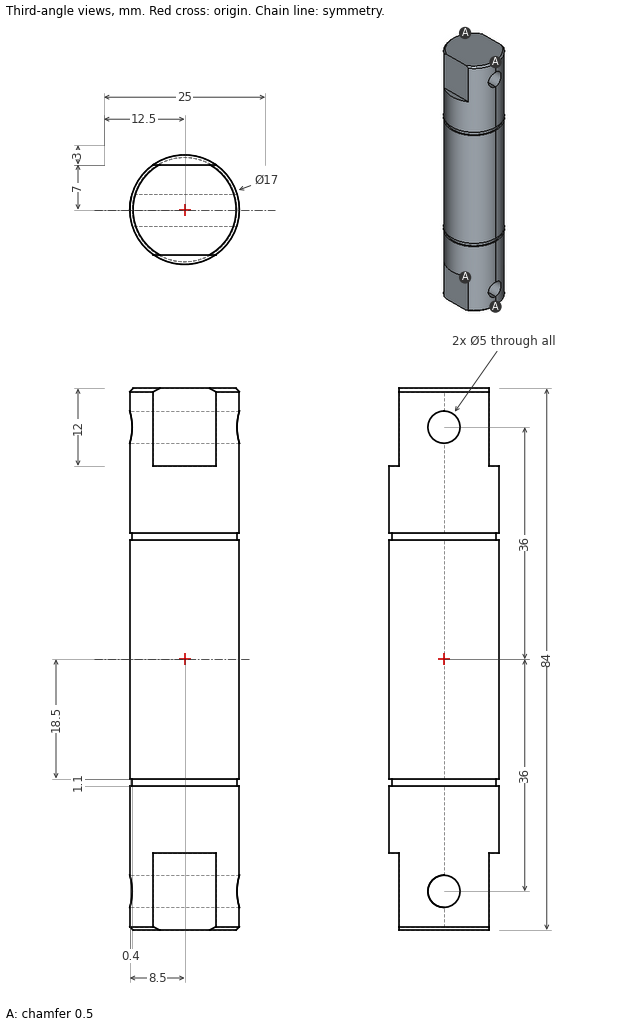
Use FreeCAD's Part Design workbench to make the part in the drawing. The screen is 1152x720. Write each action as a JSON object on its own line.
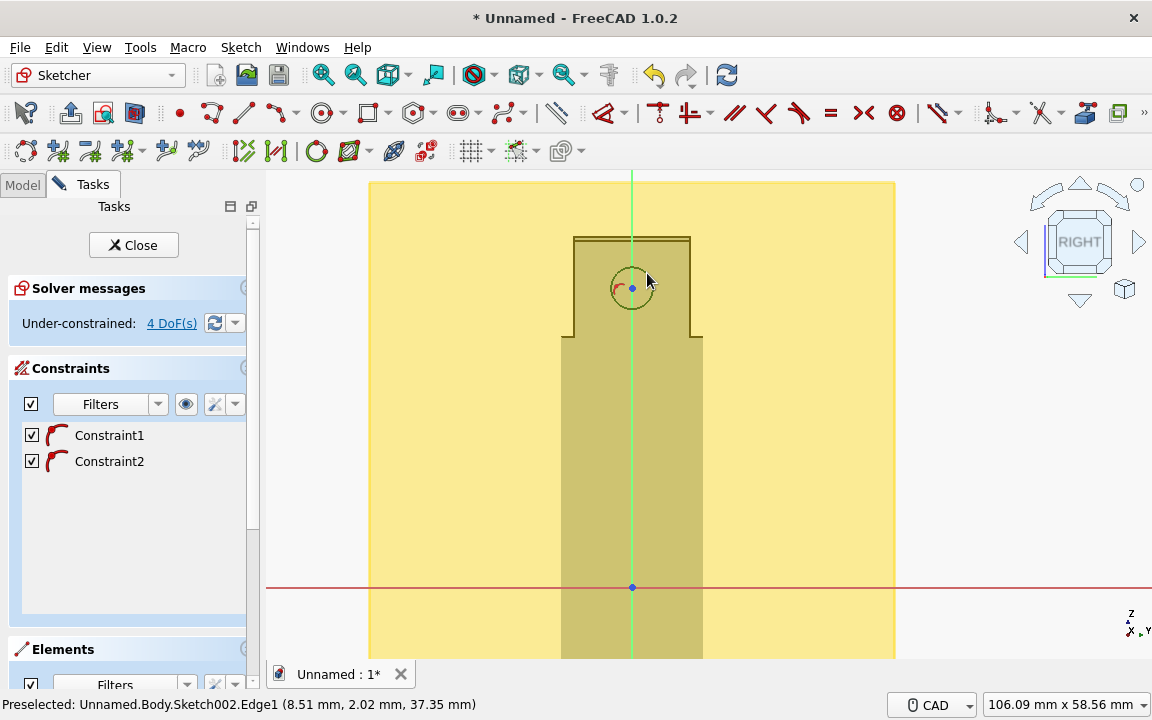
{"action": "scroll", "coordinate": [647, 273], "scroll_direction": "down", "scroll_amount": 4}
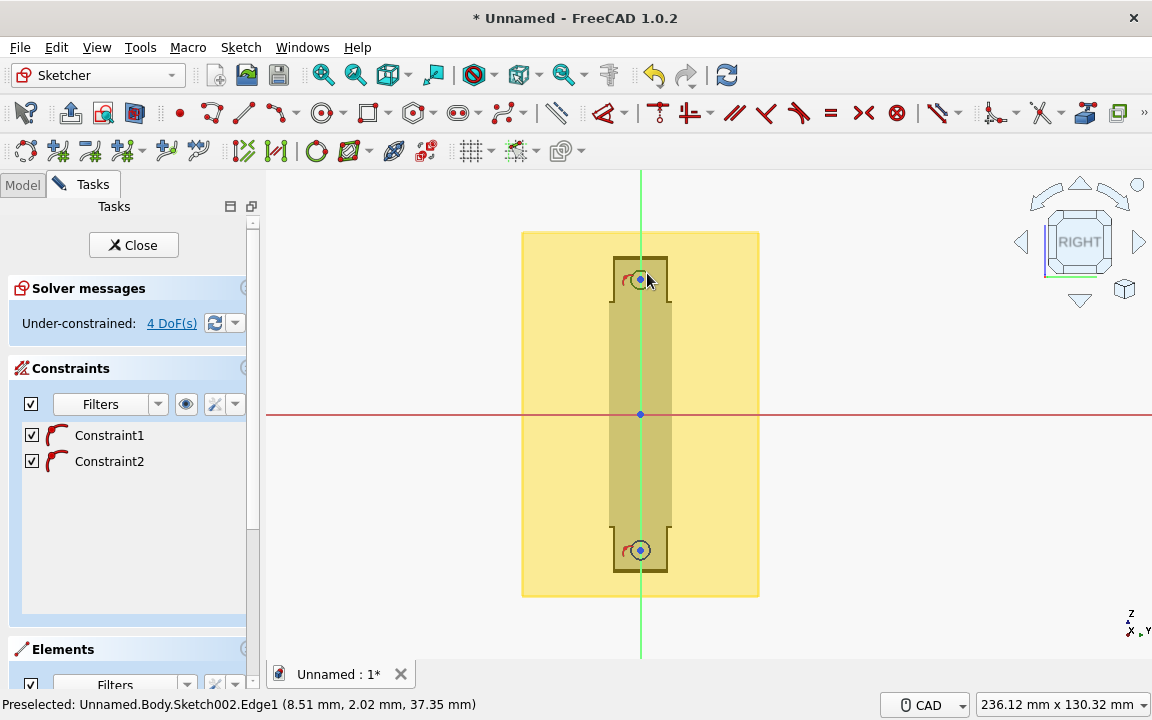
{"action": "scroll", "coordinate": [647, 544], "scroll_direction": "up", "scroll_amount": 4}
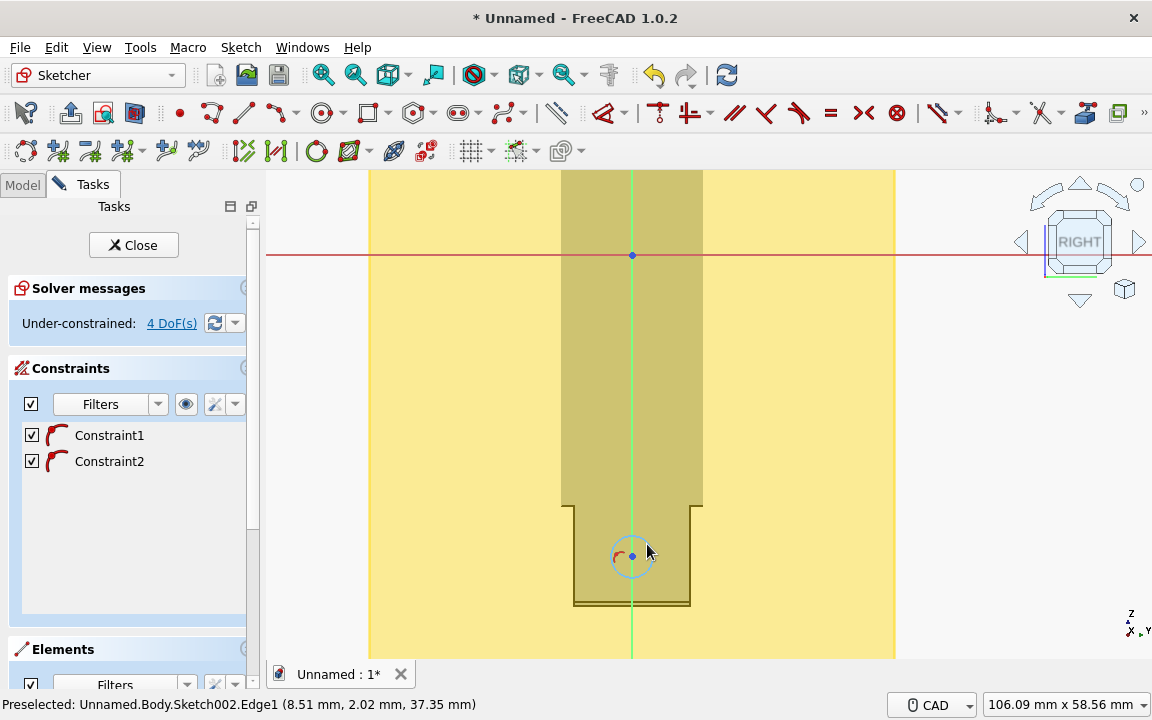
{"action": "left_click", "coordinate": [647, 542]}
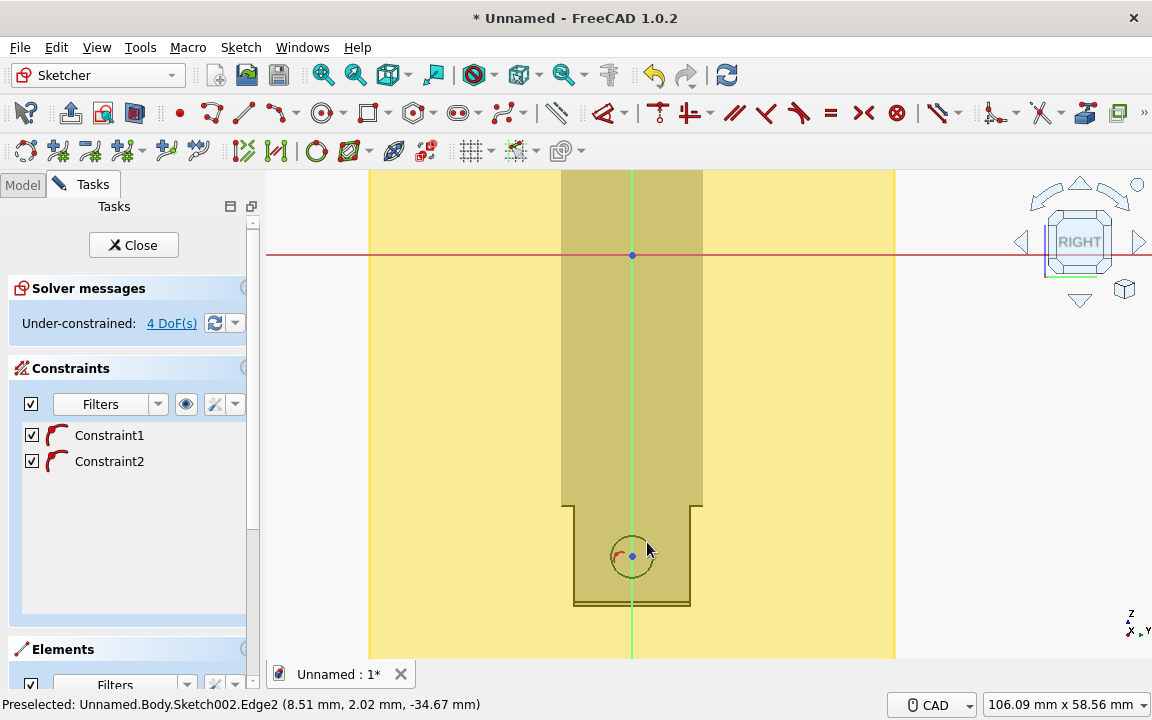
{"action": "left_click", "coordinate": [832, 114]}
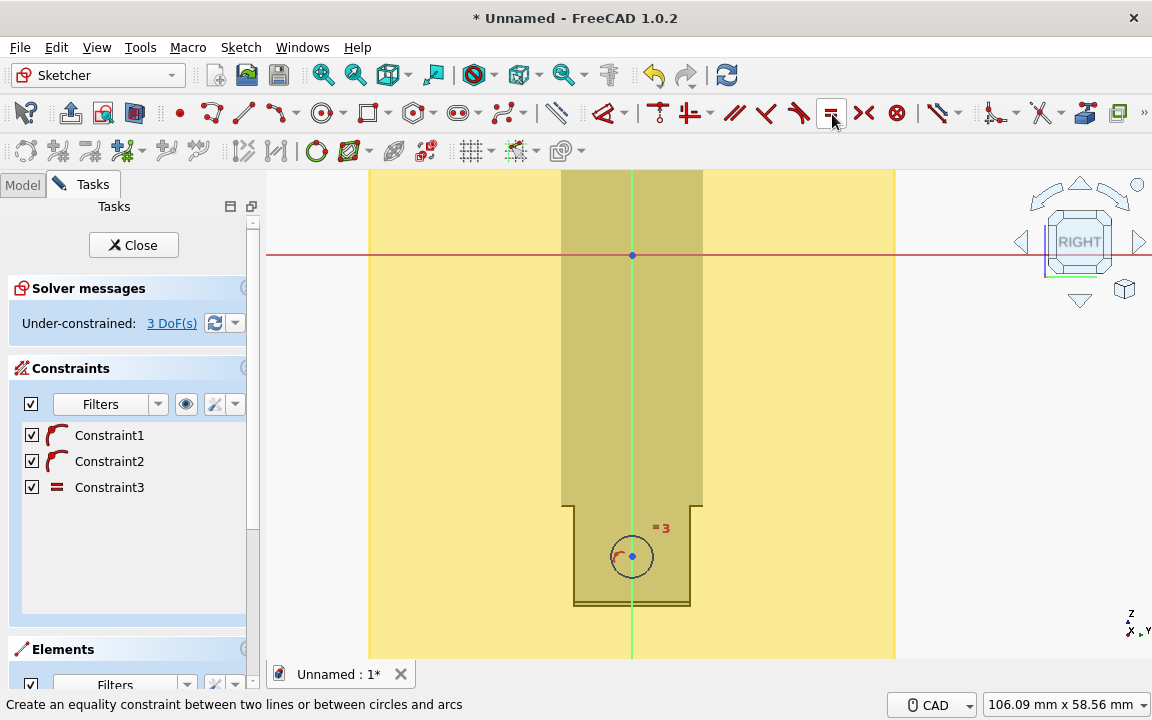
{"action": "left_click", "coordinate": [604, 114]}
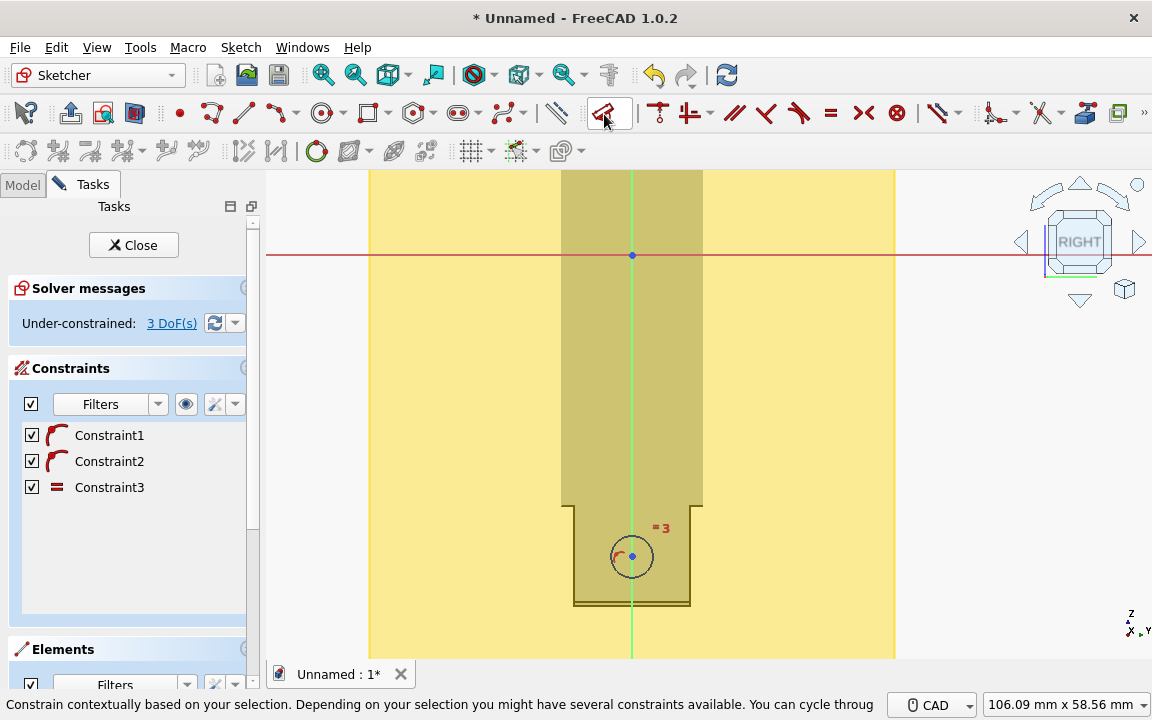
{"action": "scroll", "coordinate": [647, 545], "scroll_direction": "down", "scroll_amount": 4}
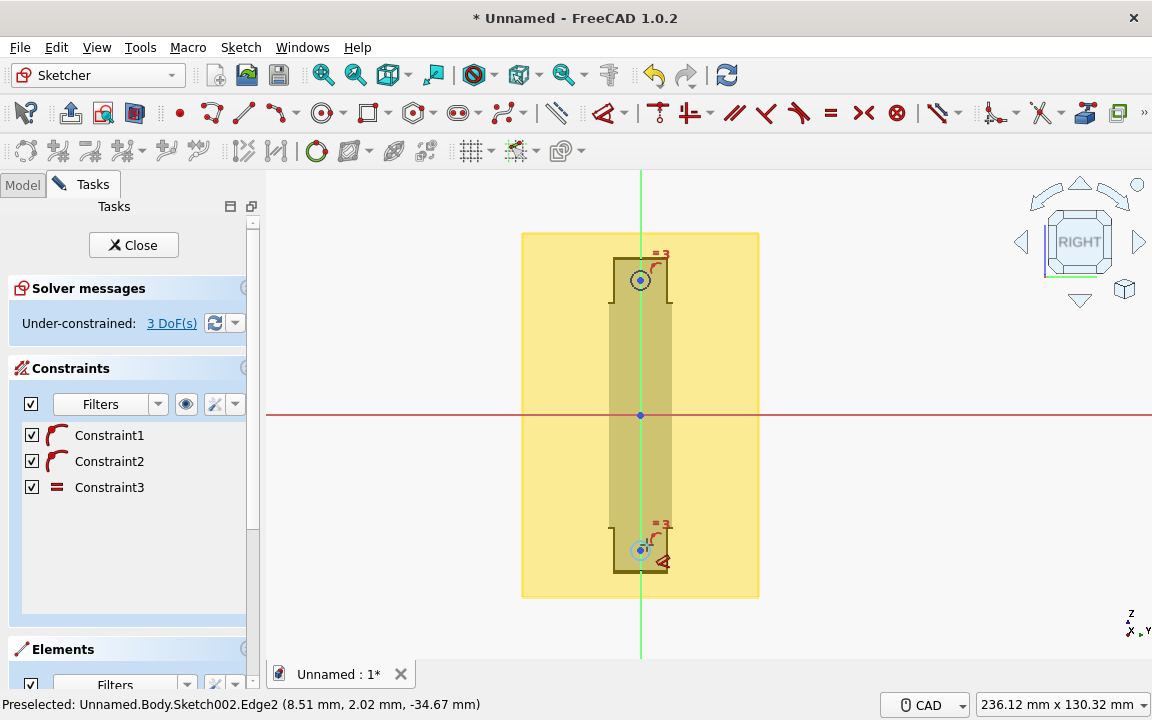
{"action": "scroll", "coordinate": [647, 274], "scroll_direction": "up", "scroll_amount": 4}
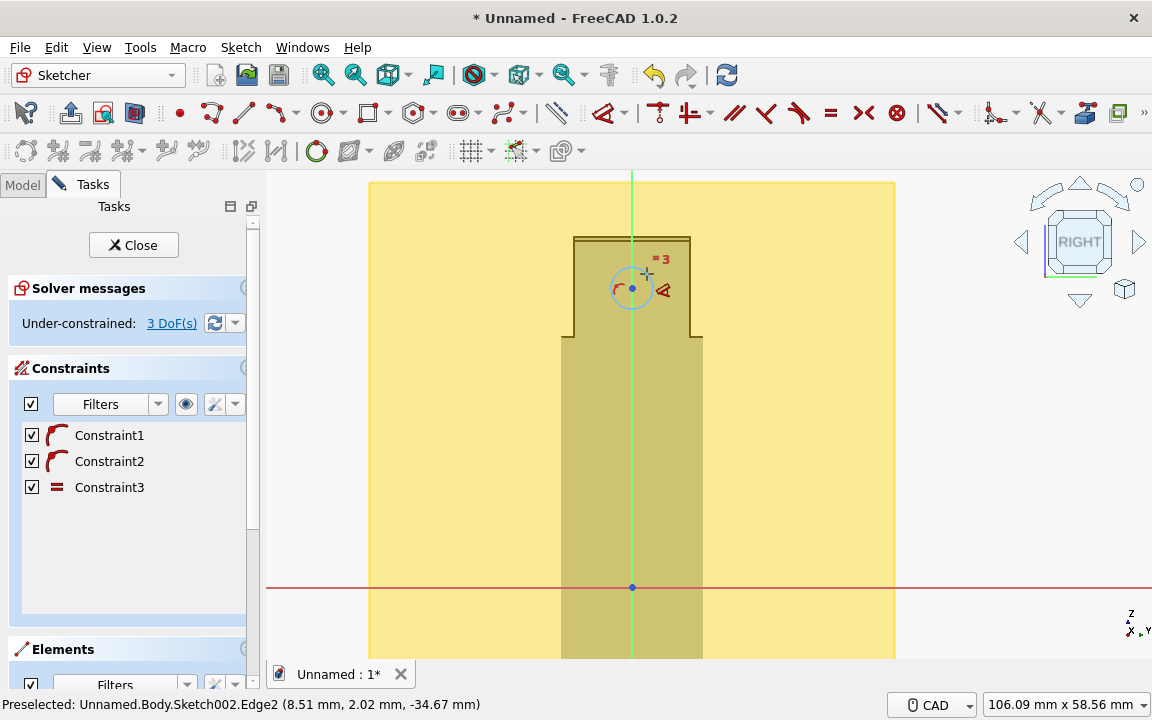
{"action": "left_click", "coordinate": [647, 273]}
{"action": "left_click", "coordinate": [669, 250]}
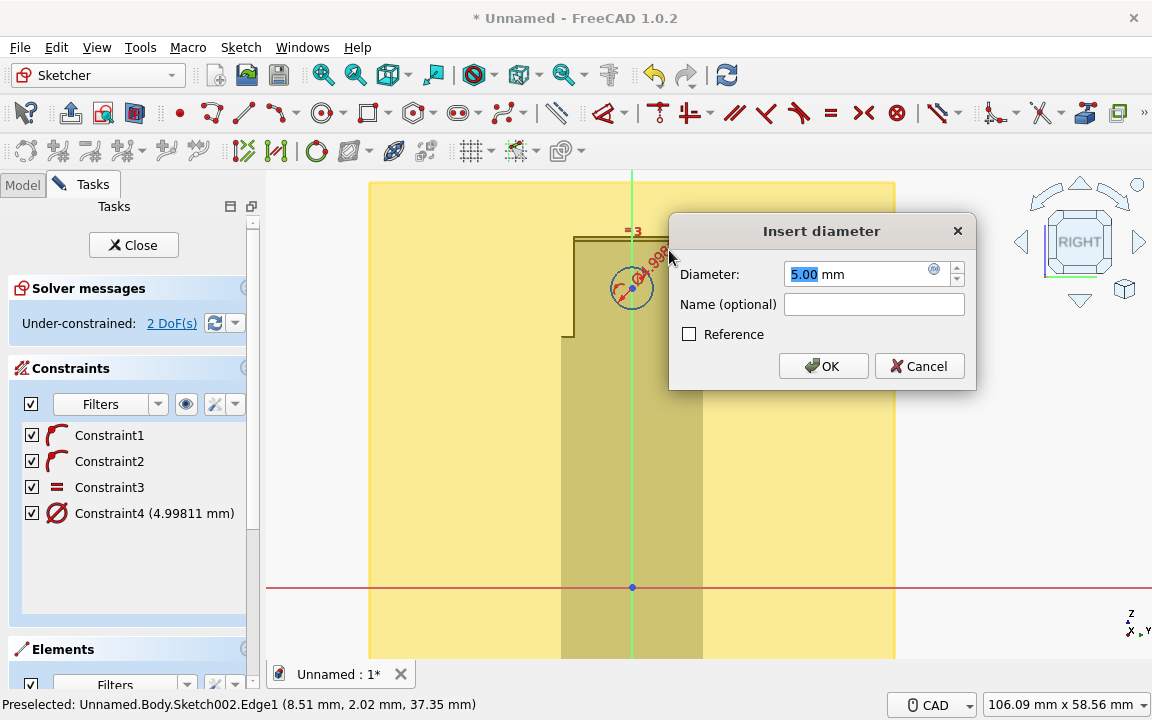
{"action": "type", "text": "5"}
{"action": "key", "text": "Return"}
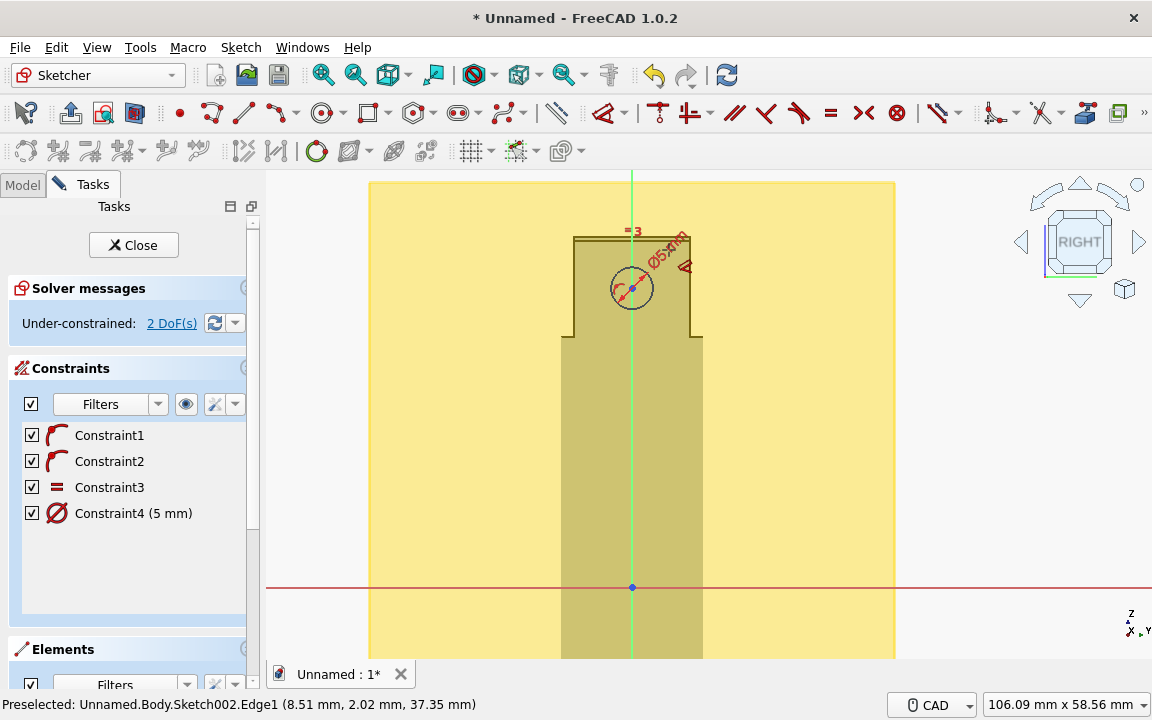
{"action": "left_click", "coordinate": [632, 288]}
{"action": "left_click", "coordinate": [666, 438]}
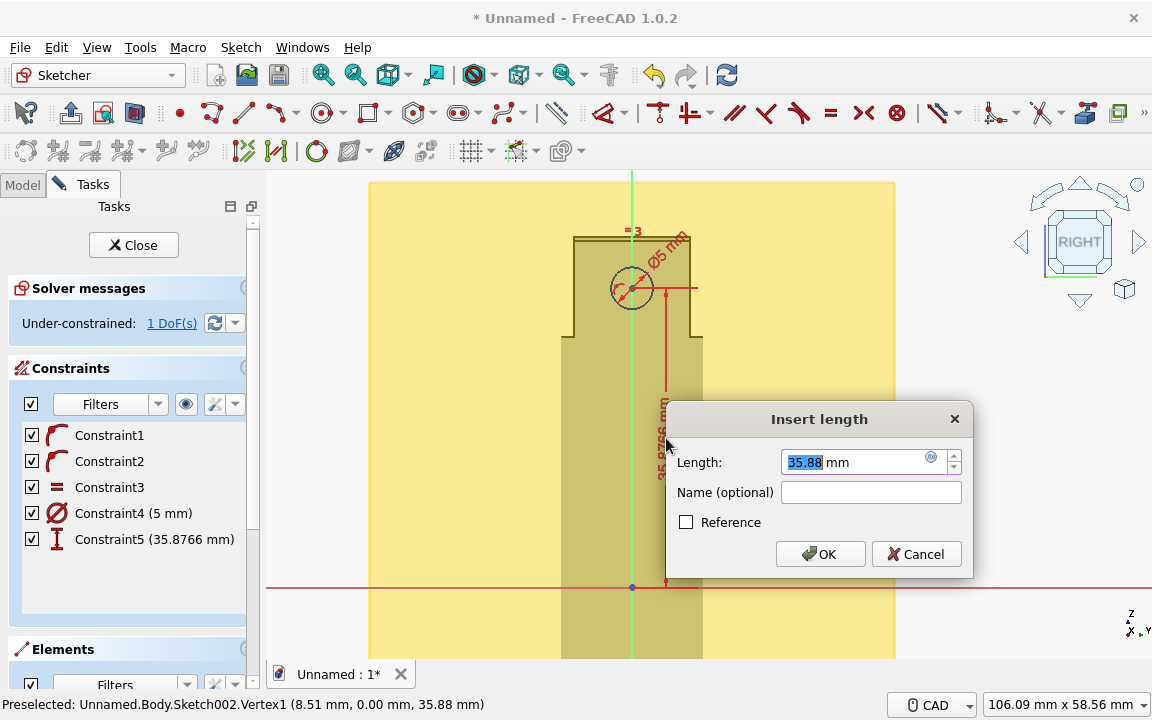
{"action": "type", "text": "36"}
{"action": "key", "text": "Return"}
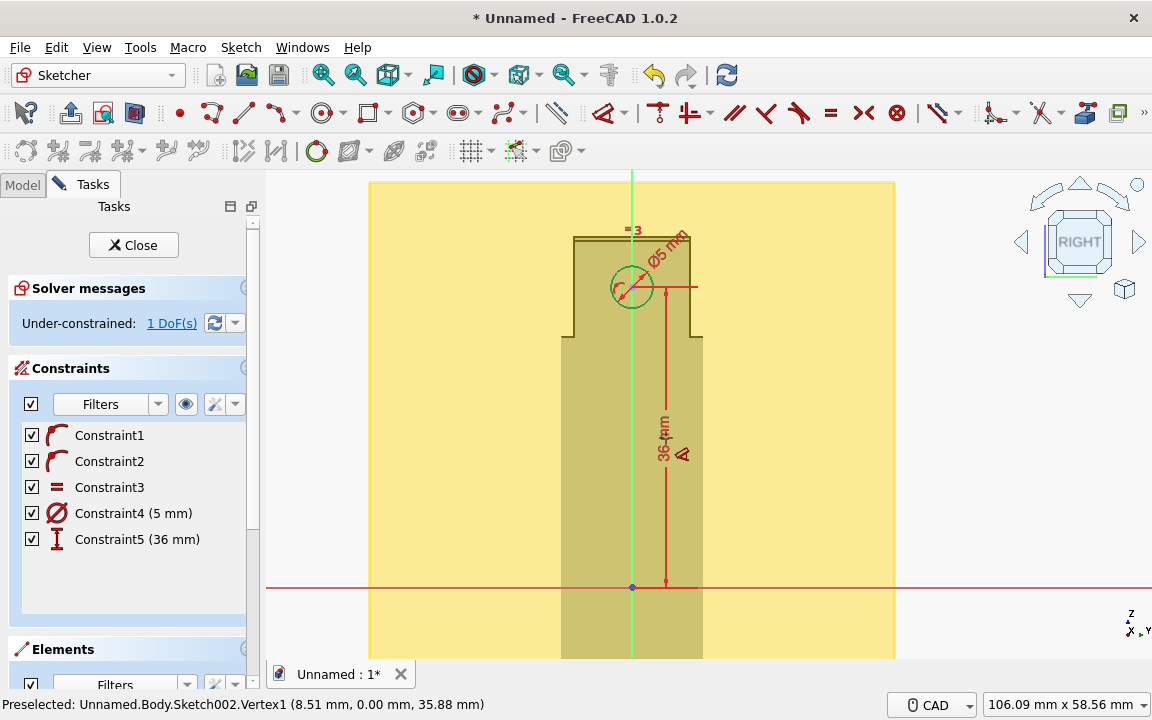
{"action": "scroll", "coordinate": [647, 273], "scroll_direction": "down", "scroll_amount": 4}